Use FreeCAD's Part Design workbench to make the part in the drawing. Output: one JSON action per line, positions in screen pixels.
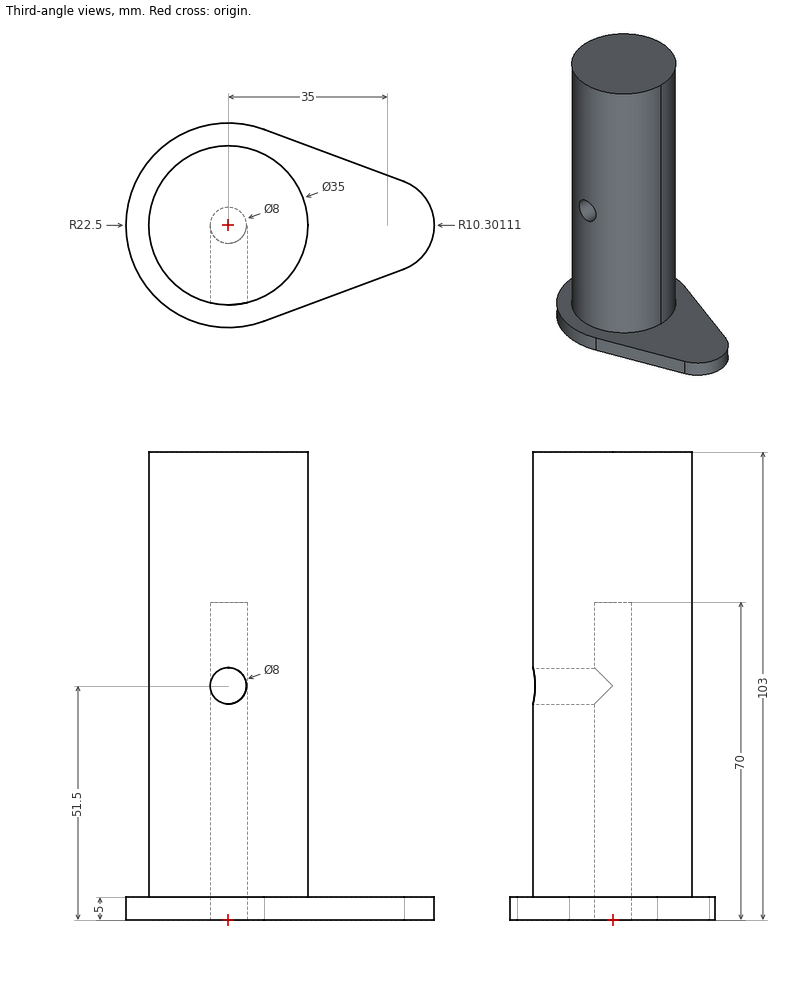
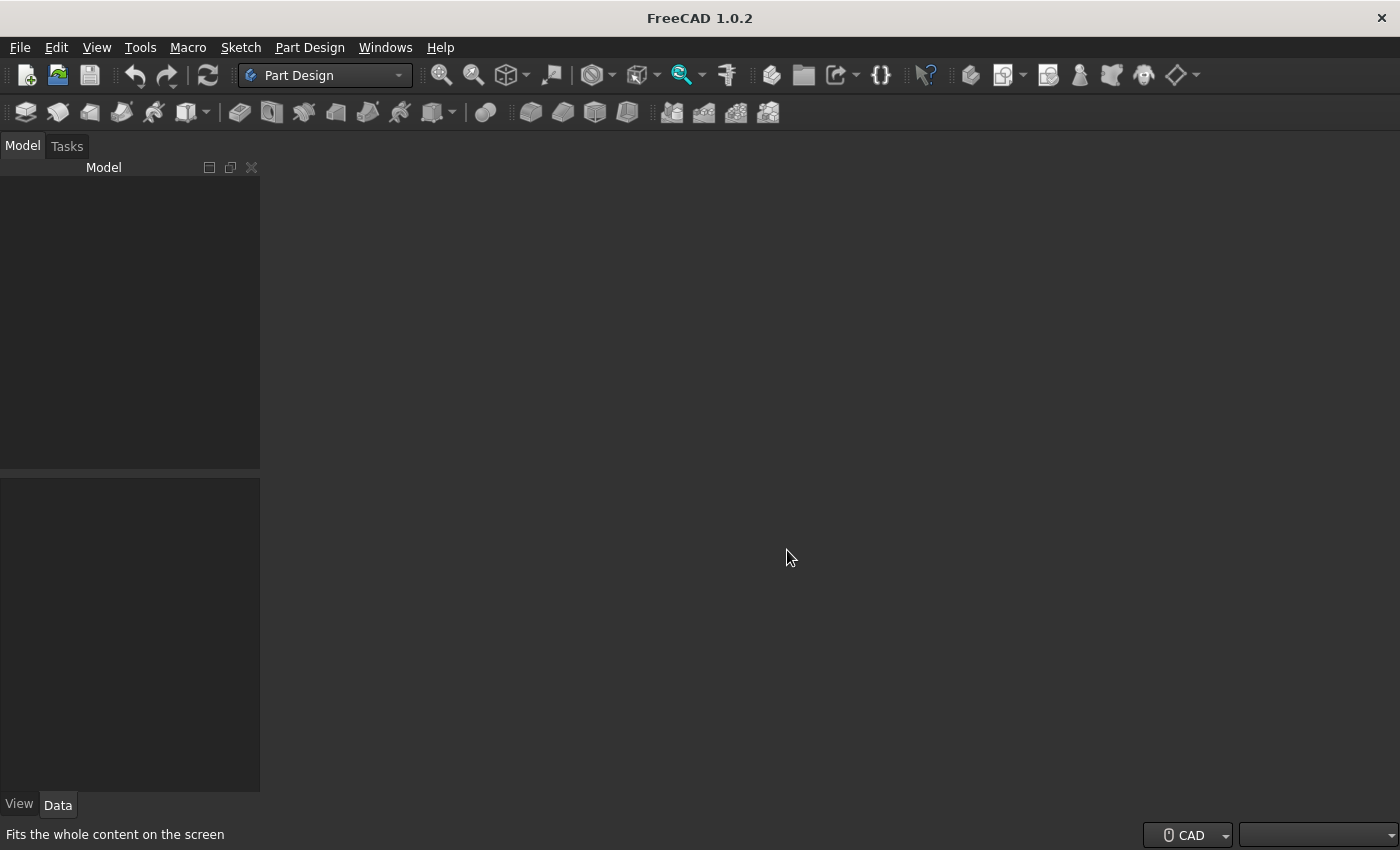
{"action": "left_click", "coordinate": [26, 76]}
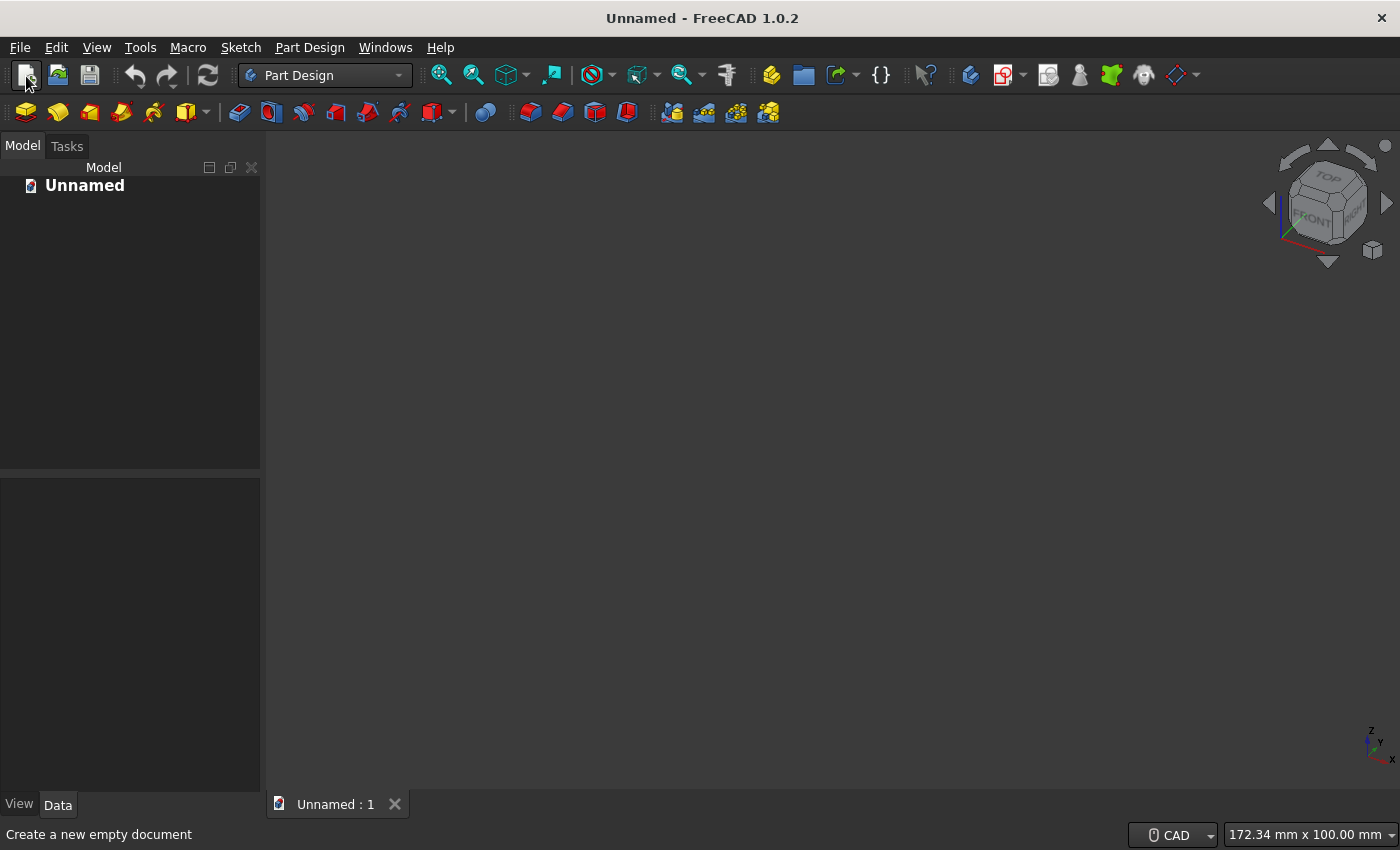
{"action": "left_click", "coordinate": [1004, 76]}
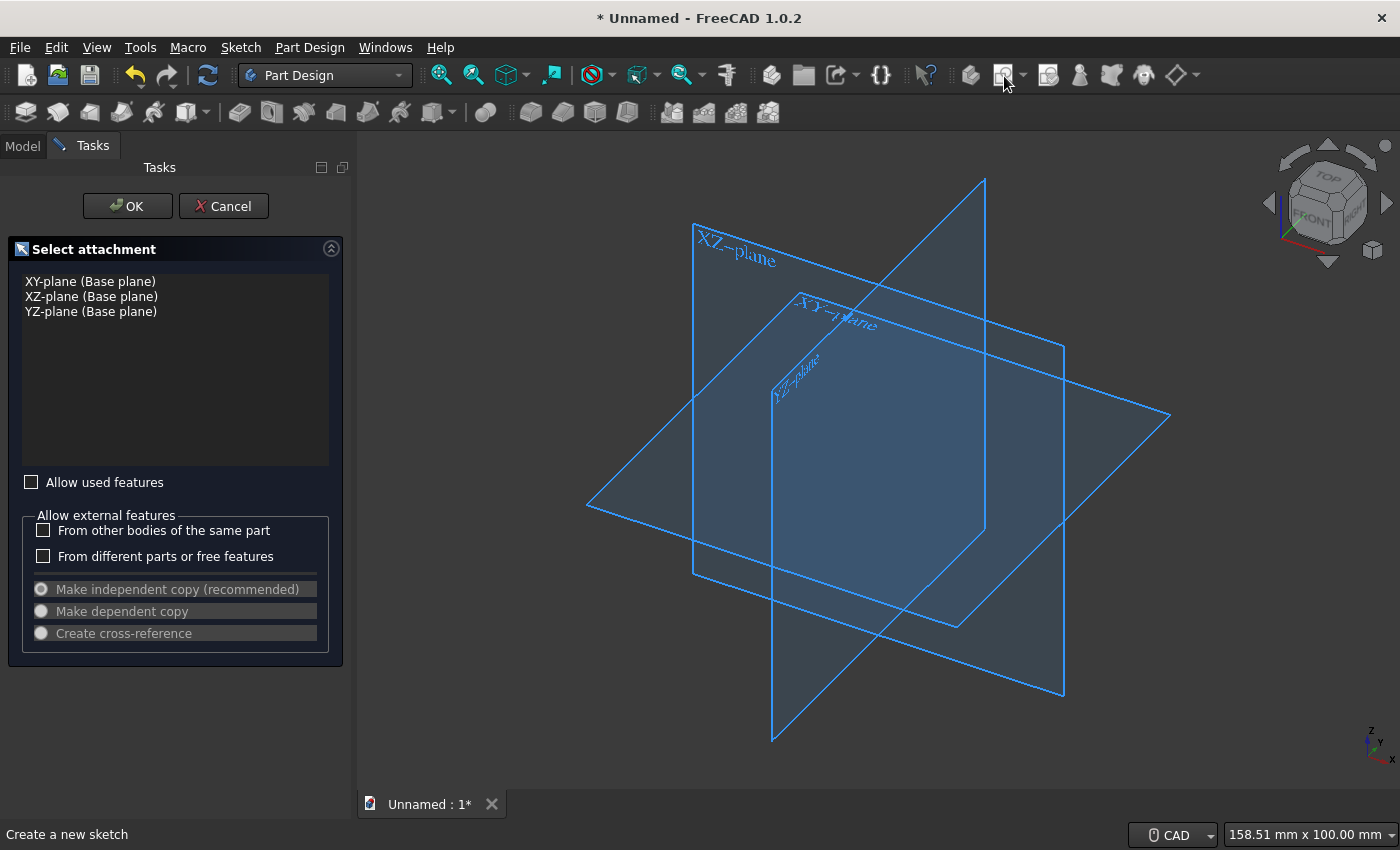
{"action": "left_click", "coordinate": [82, 282]}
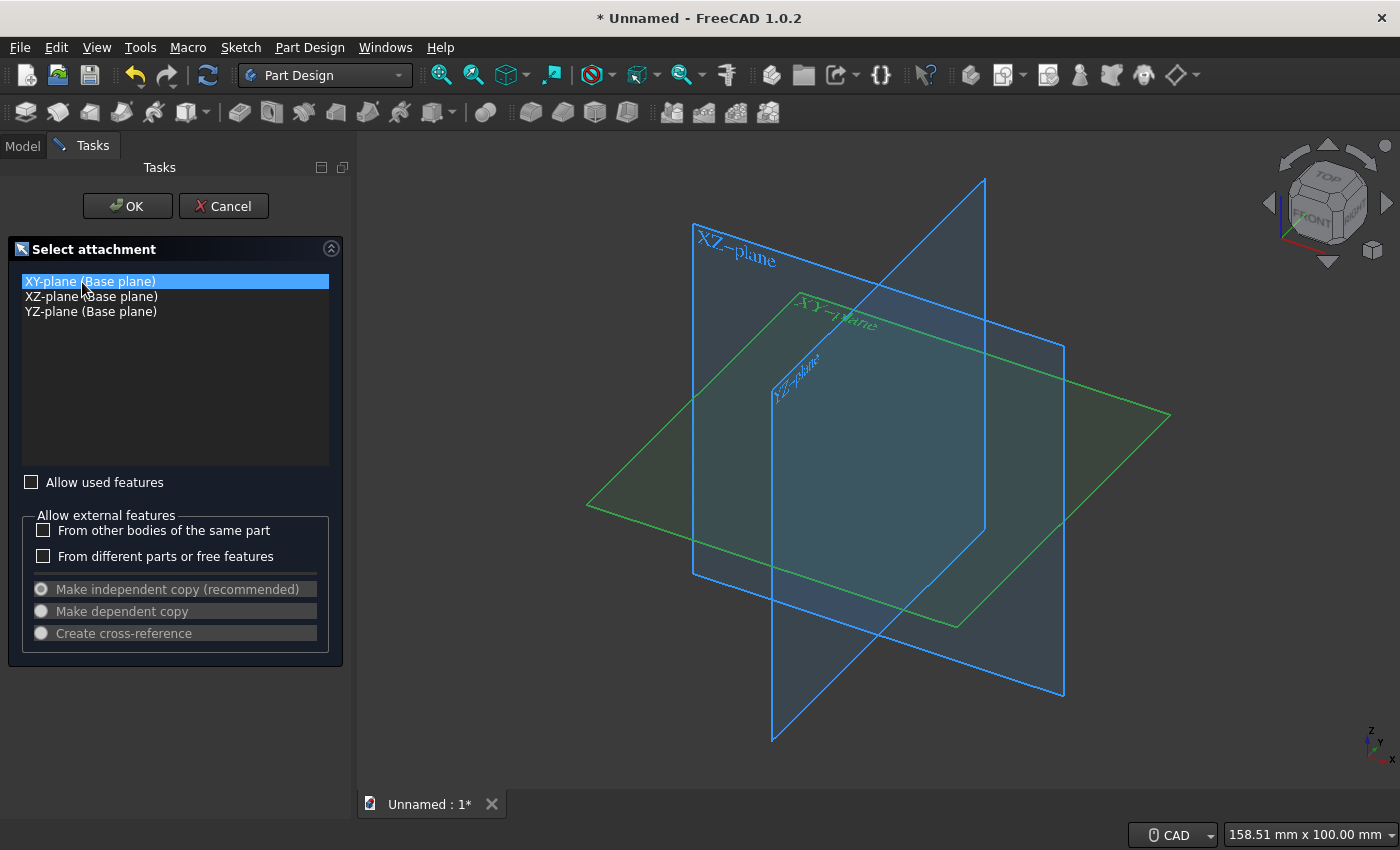
{"action": "left_click", "coordinate": [128, 206]}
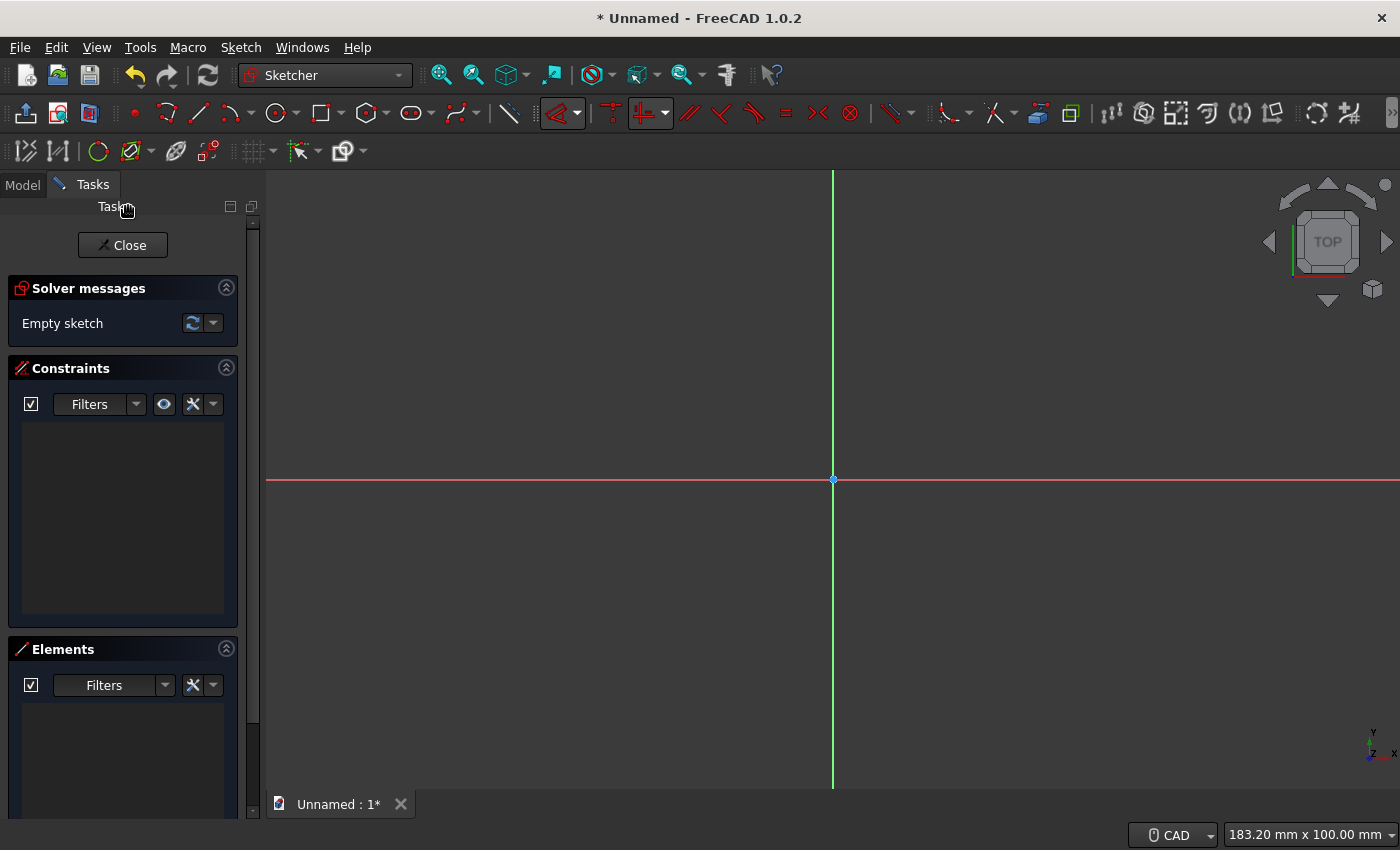
{"action": "scroll", "coordinate": [916, 480], "scroll_direction": "up", "scroll_amount": 3}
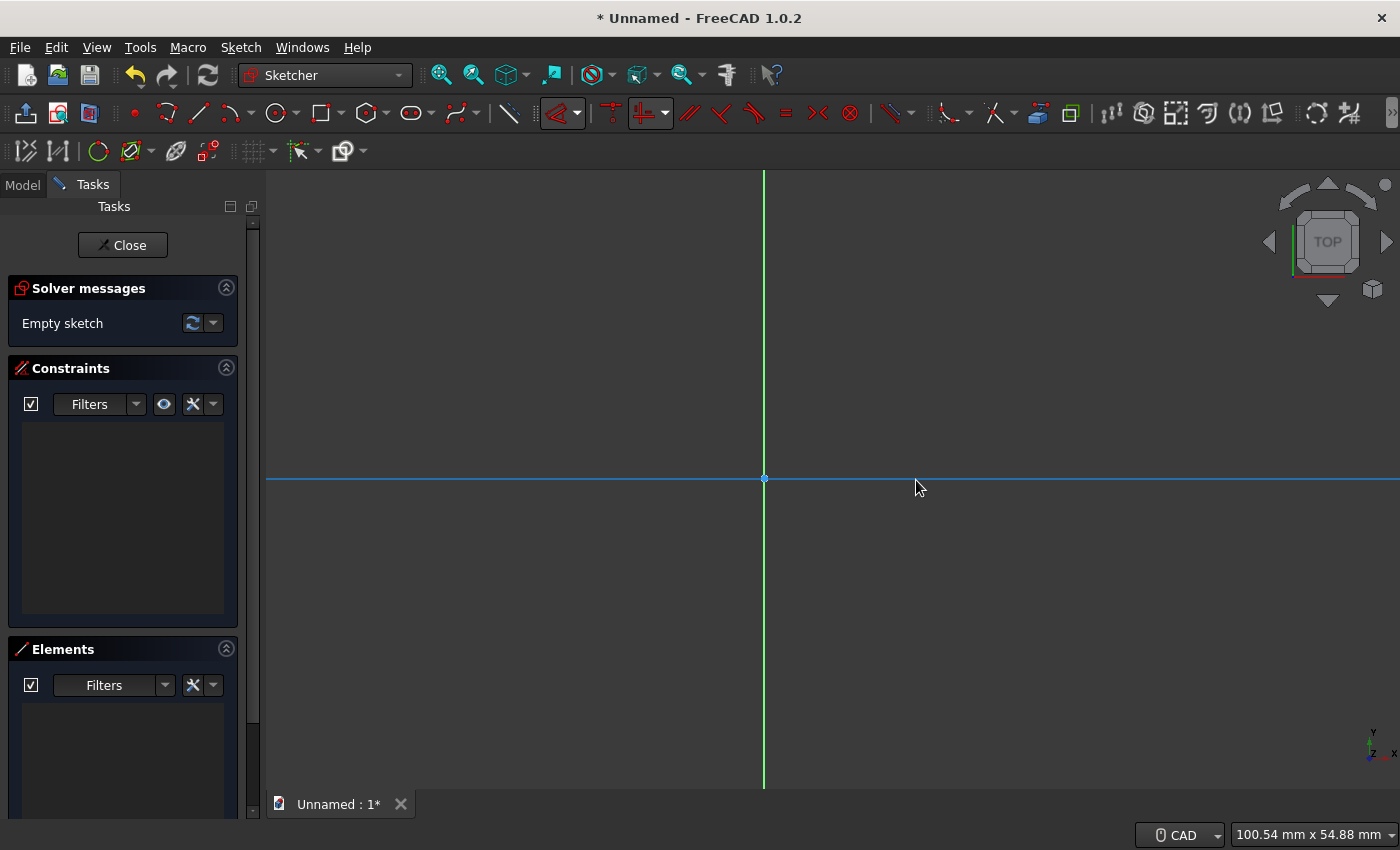
{"action": "left_click", "coordinate": [276, 114]}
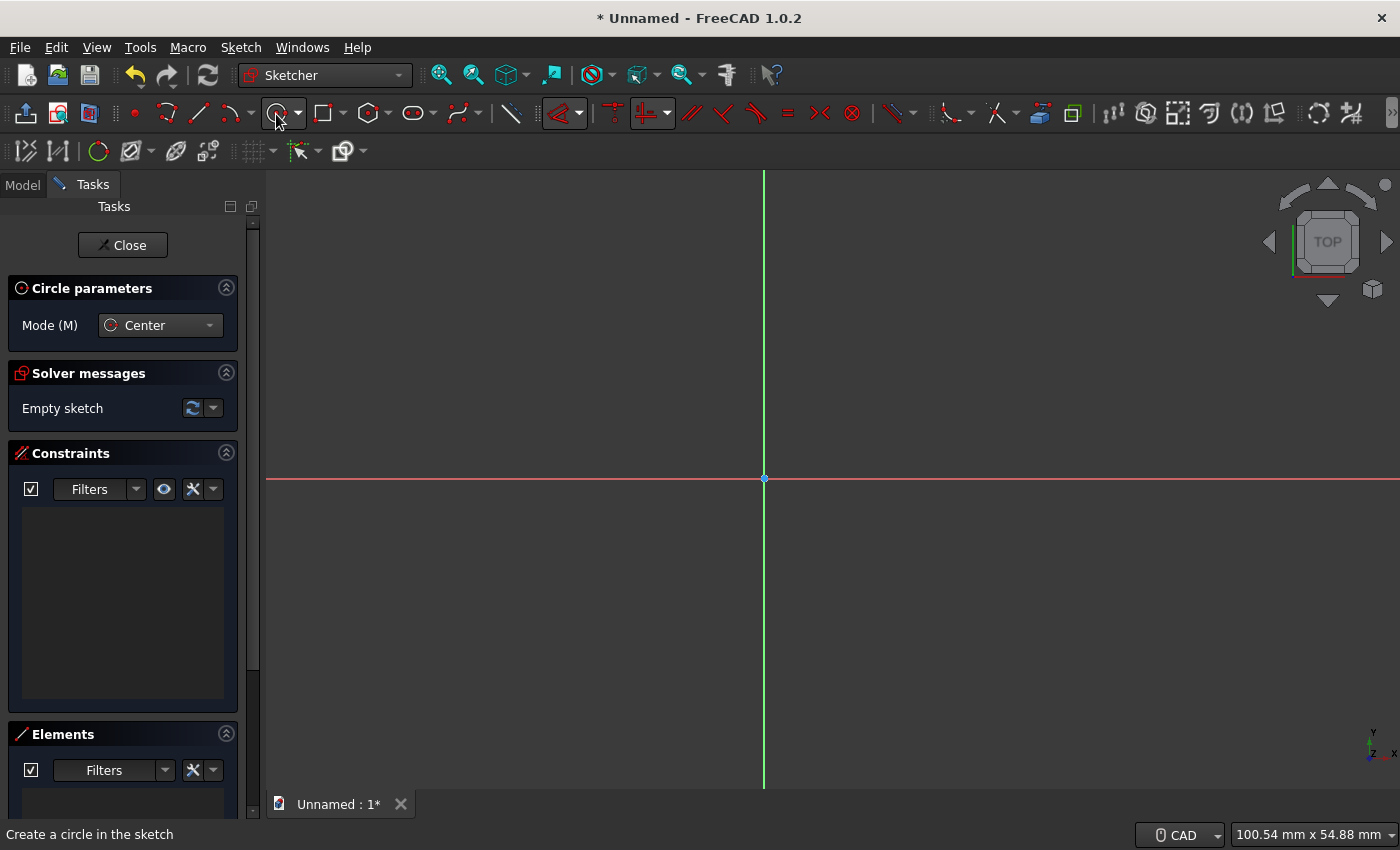
{"action": "left_click", "coordinate": [764, 479]}
{"action": "left_click", "coordinate": [904, 339]}
{"action": "key", "text": "Escape"}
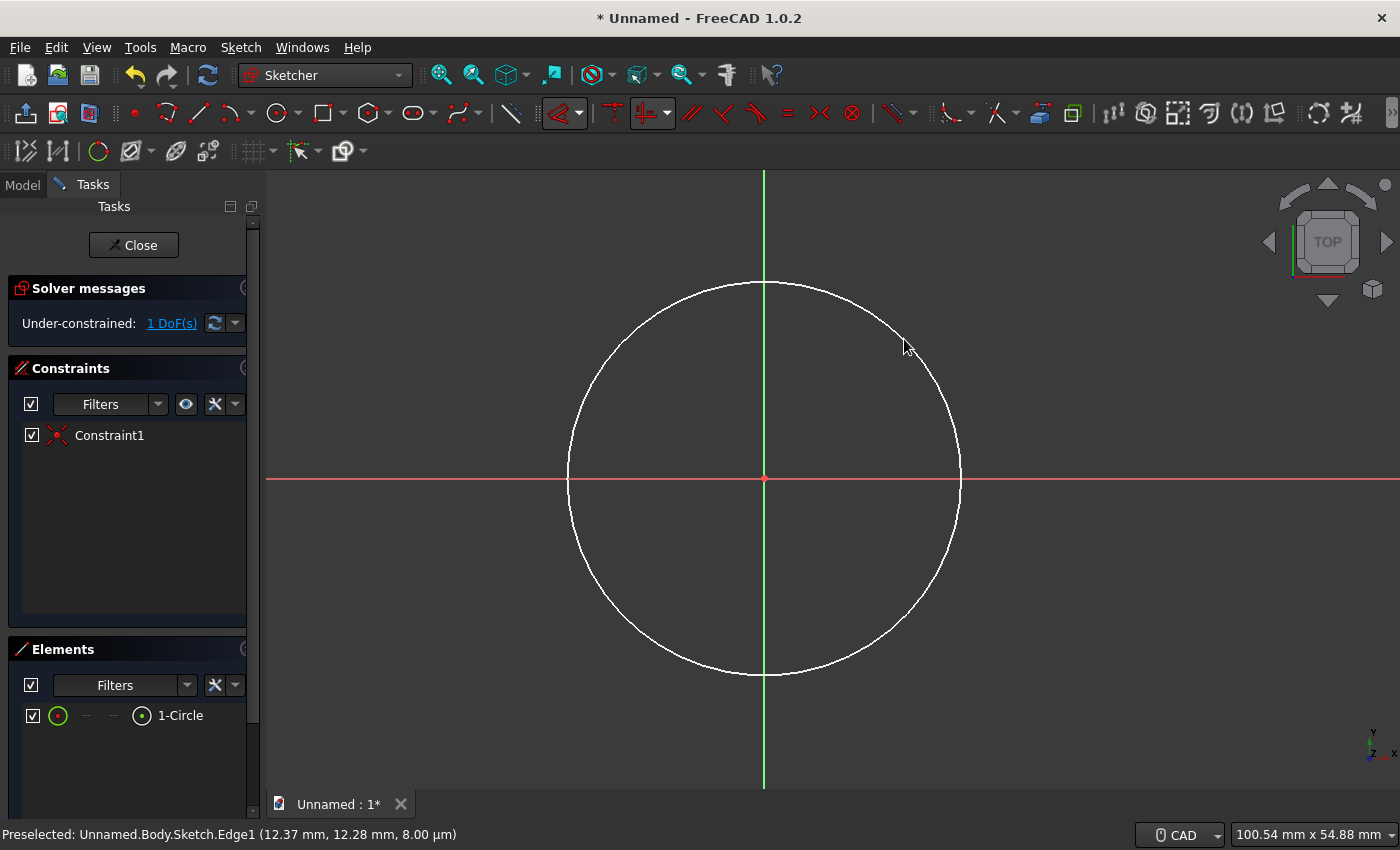
{"action": "left_click", "coordinate": [903, 339]}